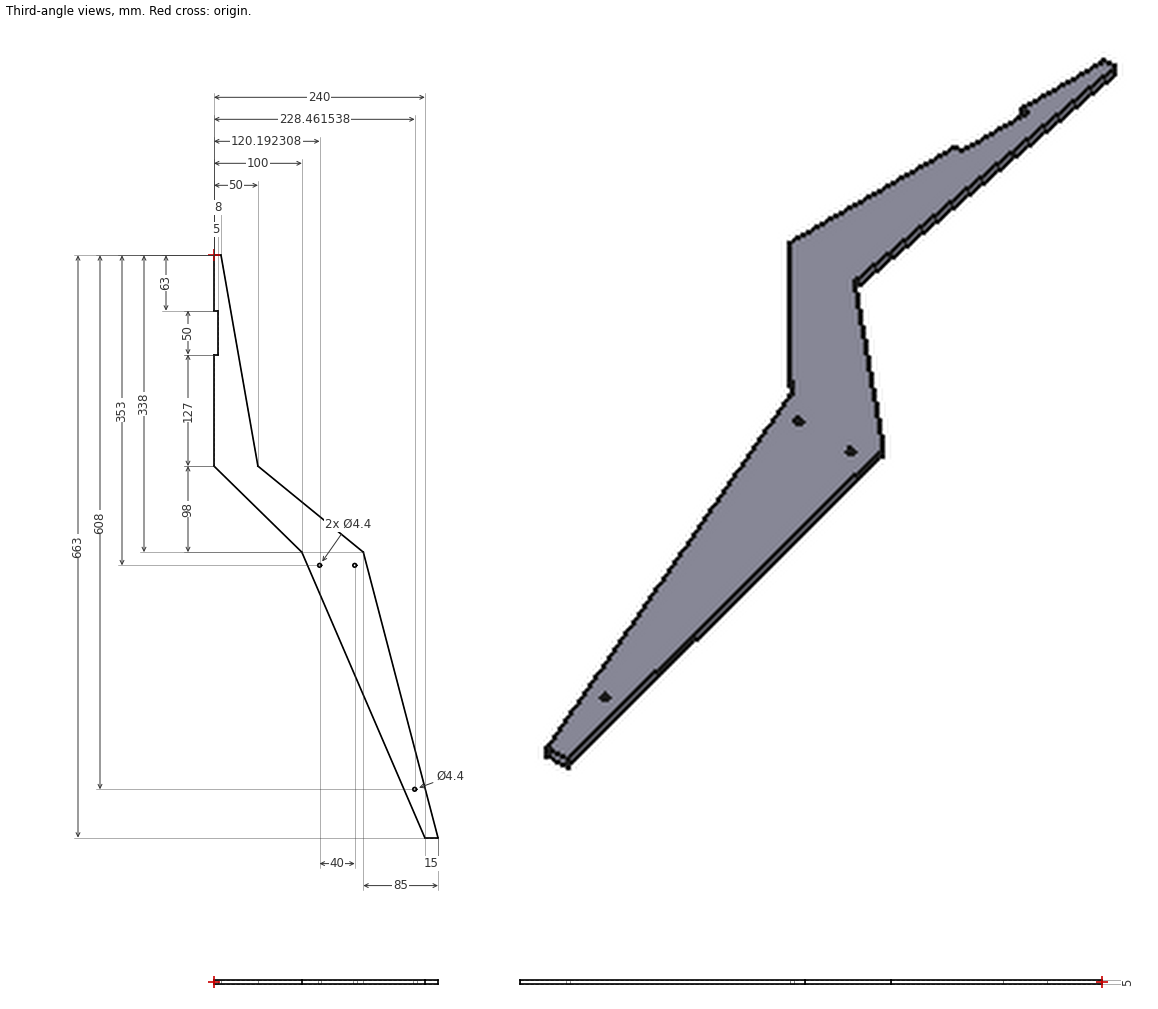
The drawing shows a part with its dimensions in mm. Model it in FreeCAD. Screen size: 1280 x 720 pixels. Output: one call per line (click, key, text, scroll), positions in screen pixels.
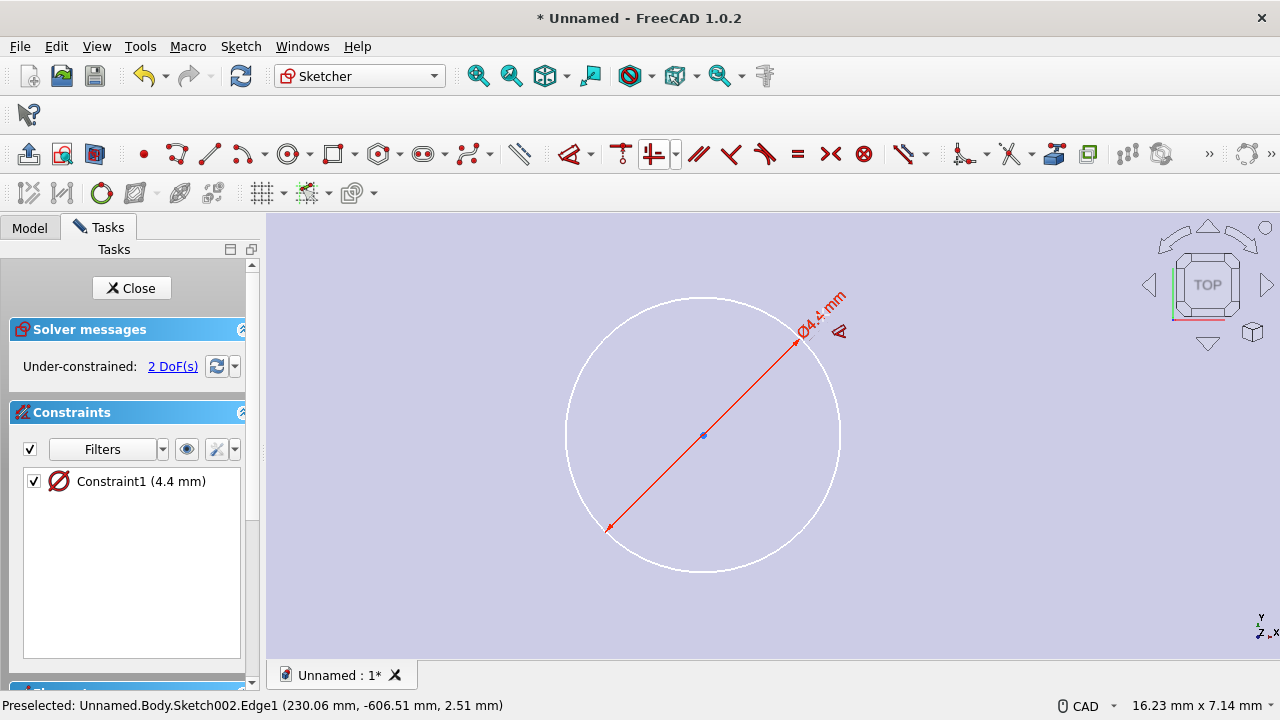
click(703, 435)
click(737, 338)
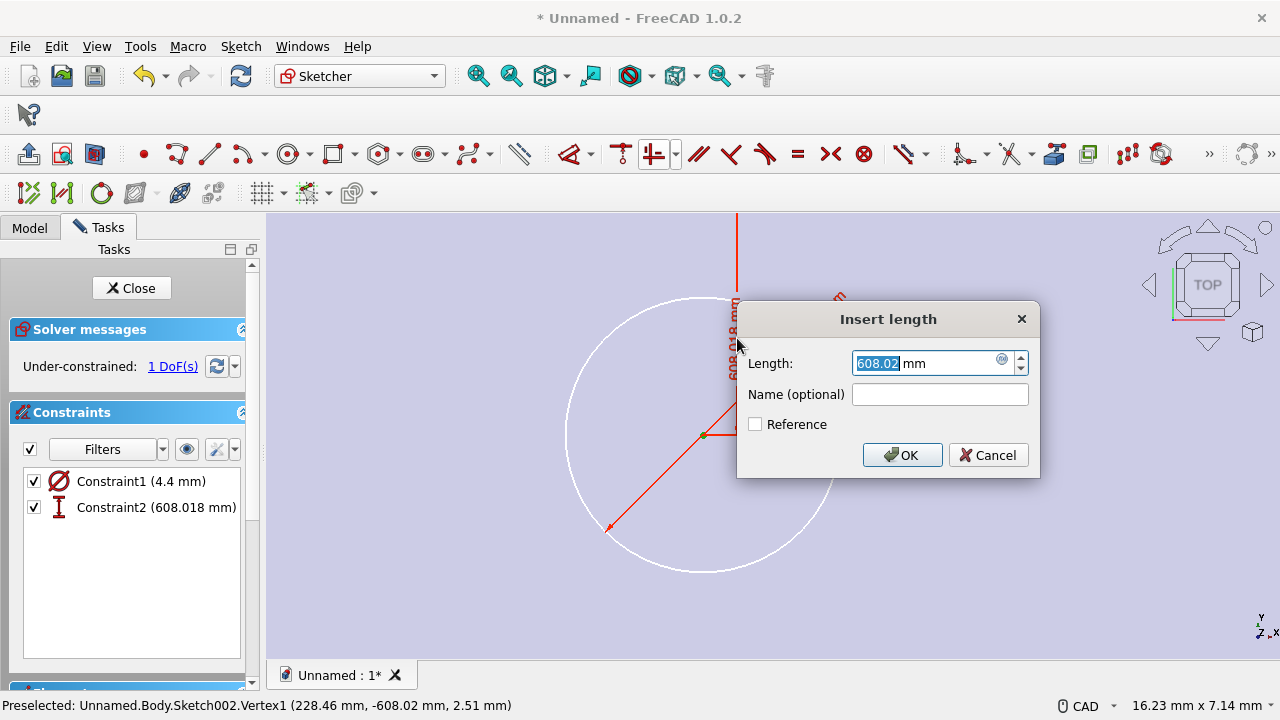
text(608)
key(Return)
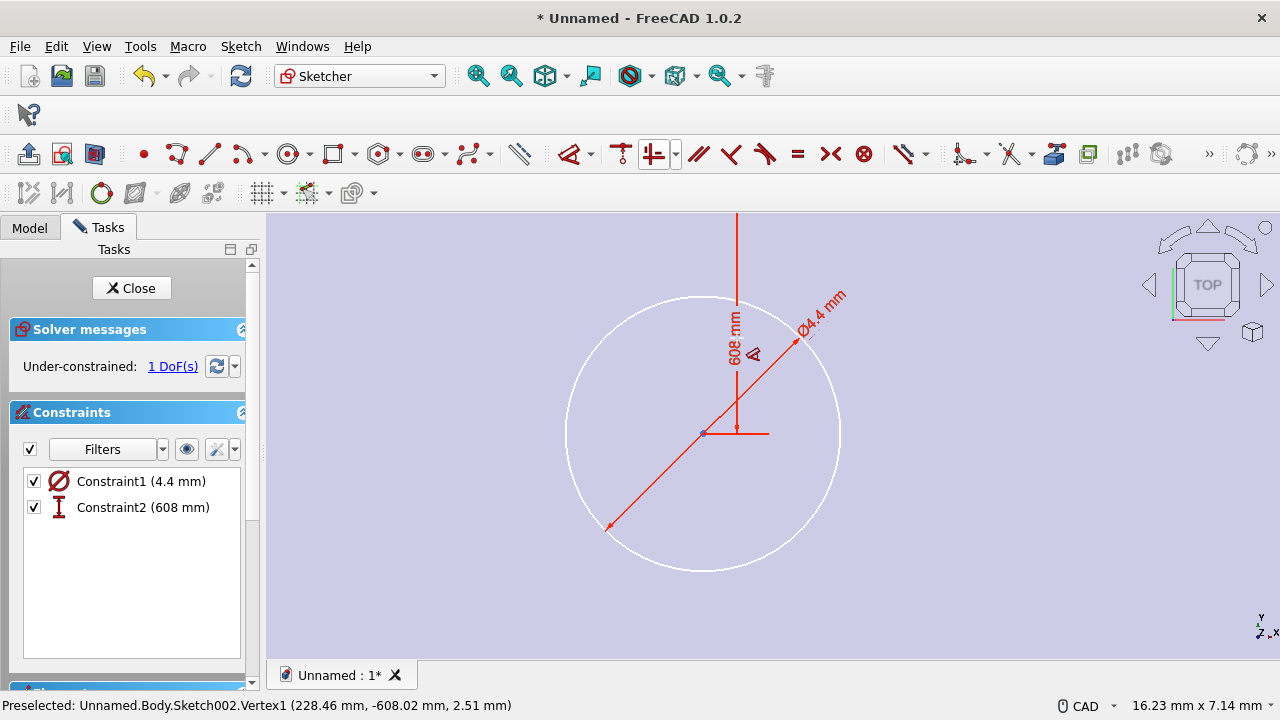
click(703, 434)
click(499, 468)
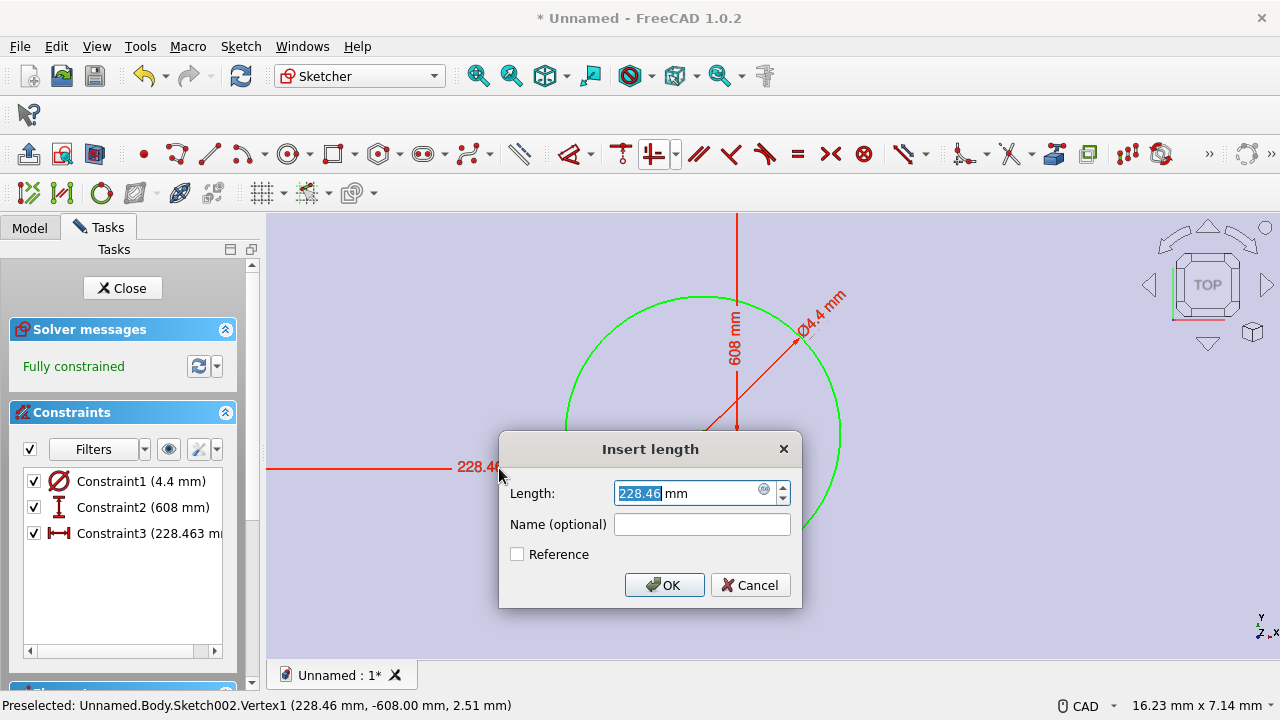
text(228.461538)
key(Return)
key(Escape)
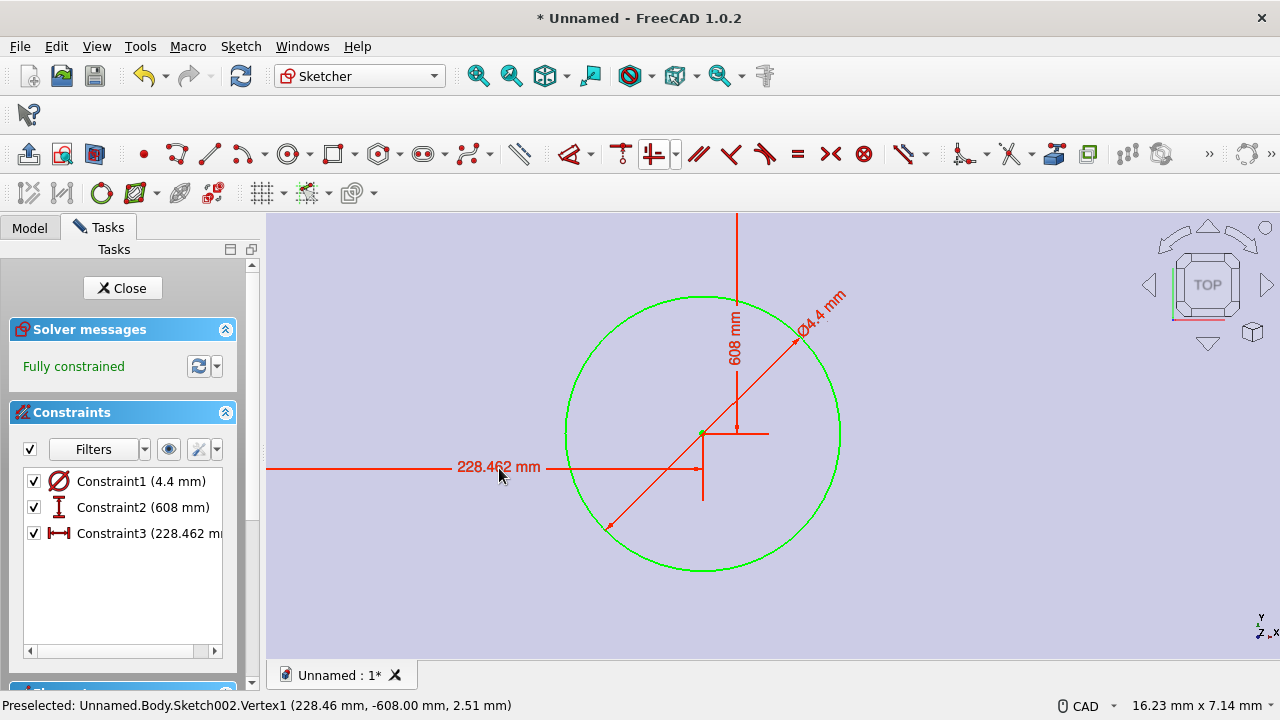
click(123, 288)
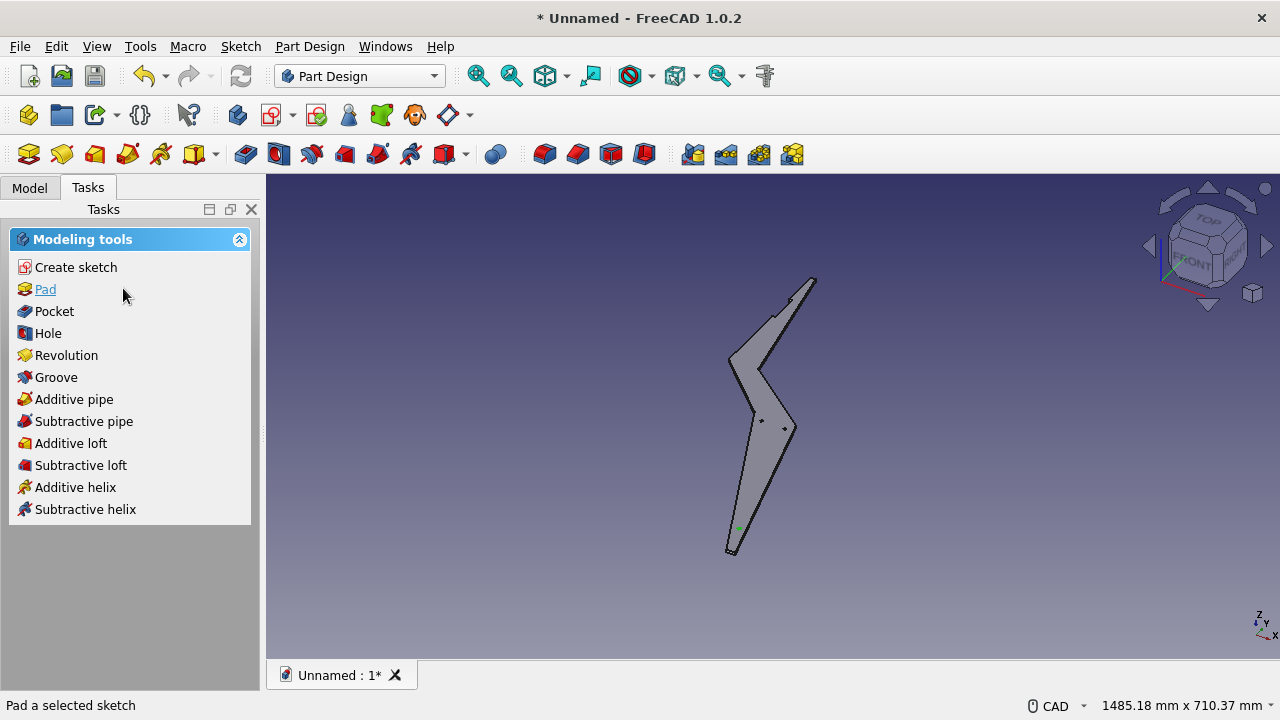
click(246, 154)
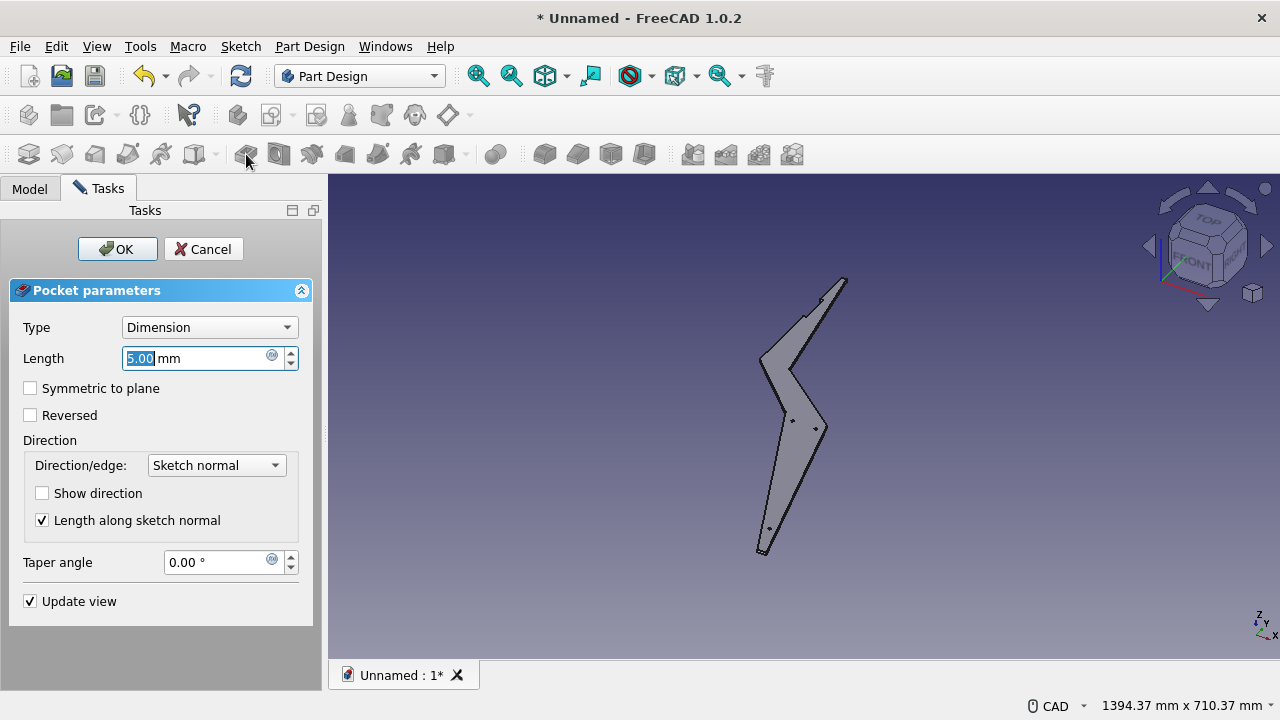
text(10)
key(Tab)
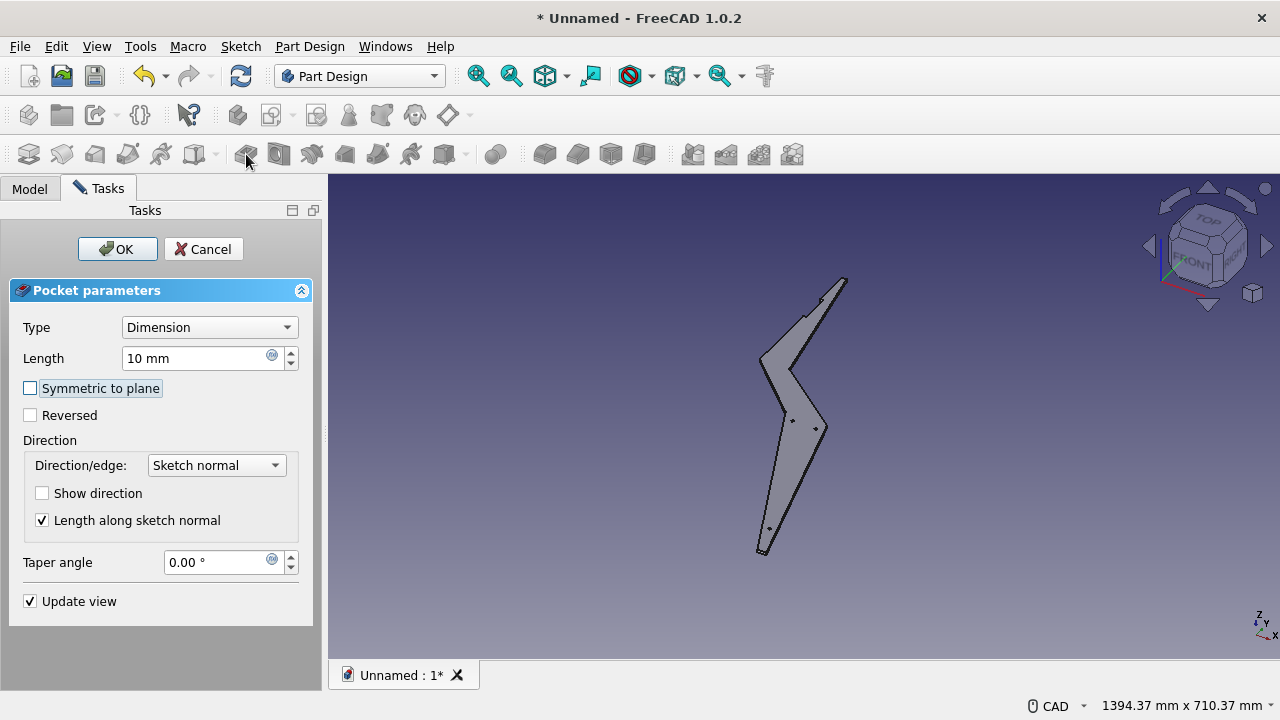
click(118, 249)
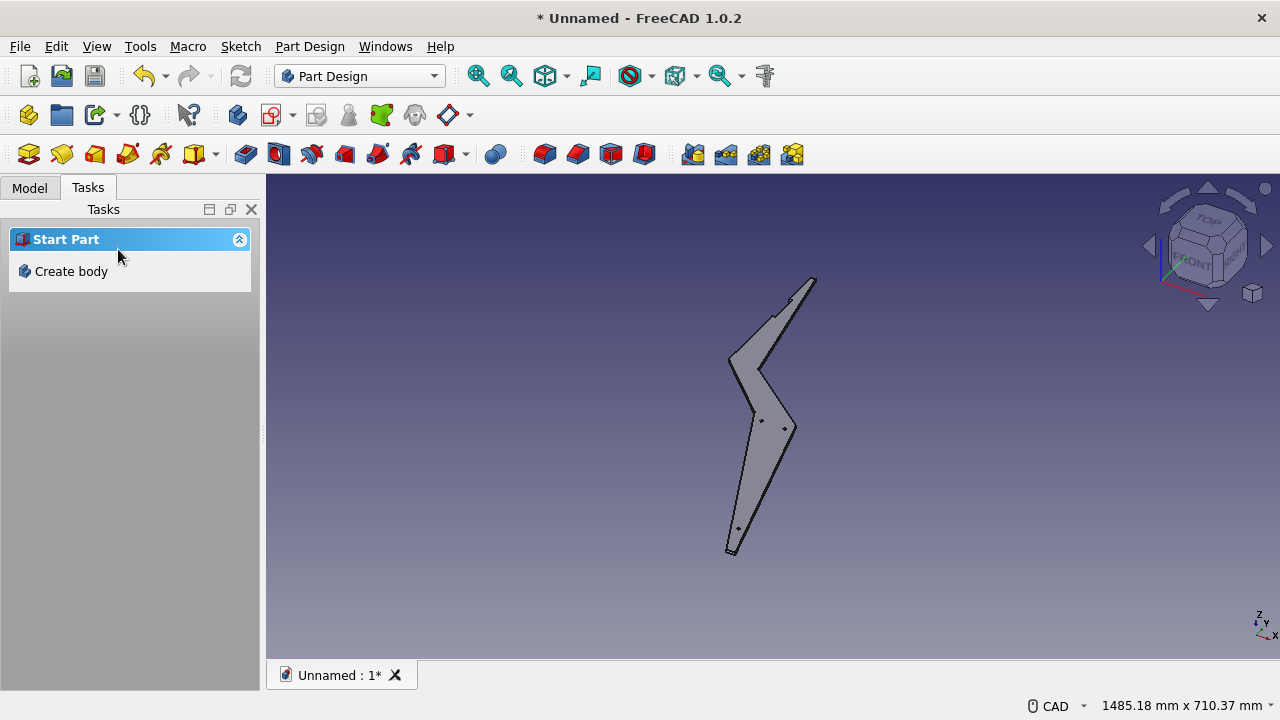
key(0)